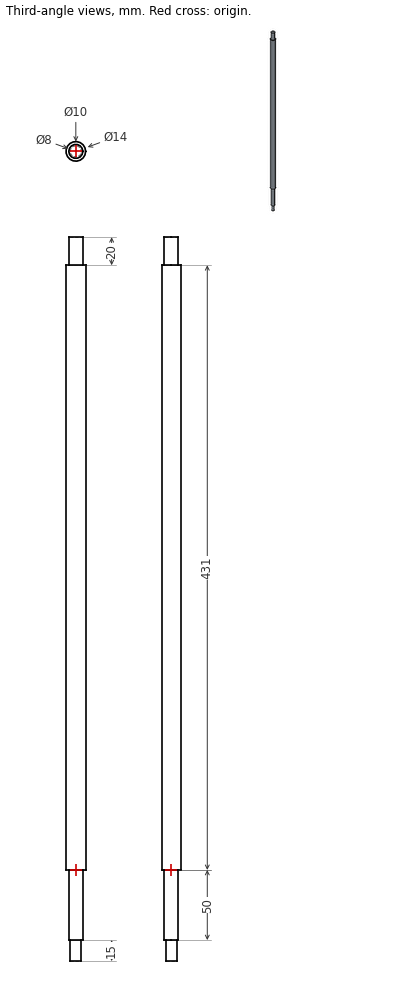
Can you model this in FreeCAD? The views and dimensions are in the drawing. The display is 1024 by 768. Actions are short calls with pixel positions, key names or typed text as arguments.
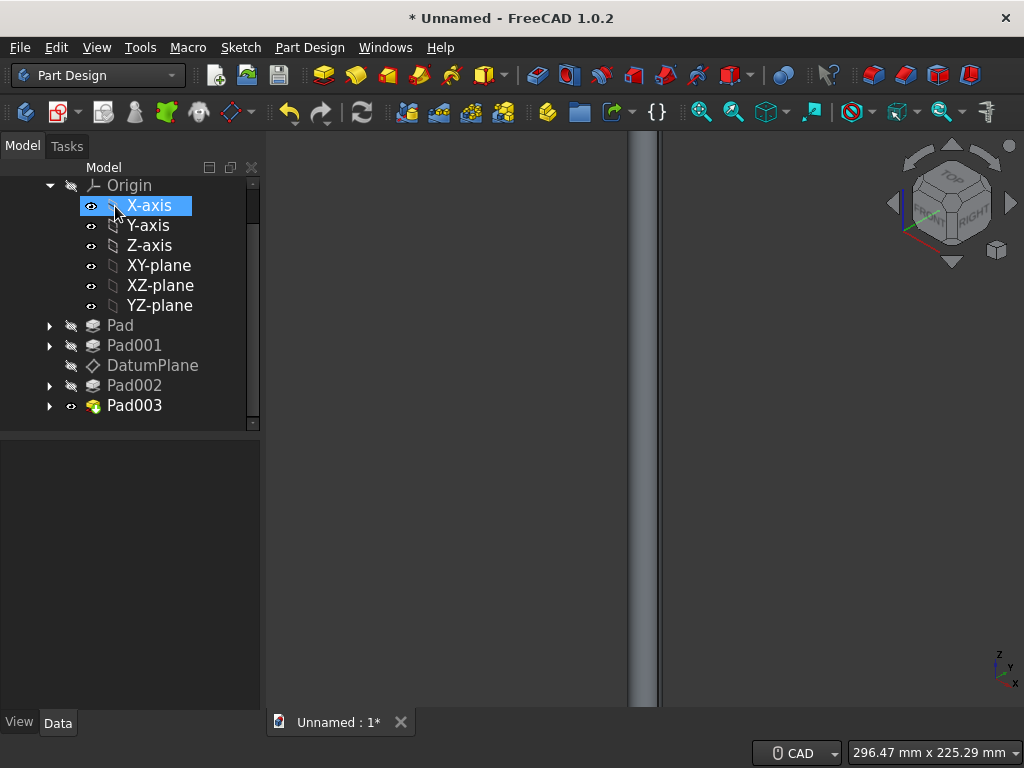
click(702, 112)